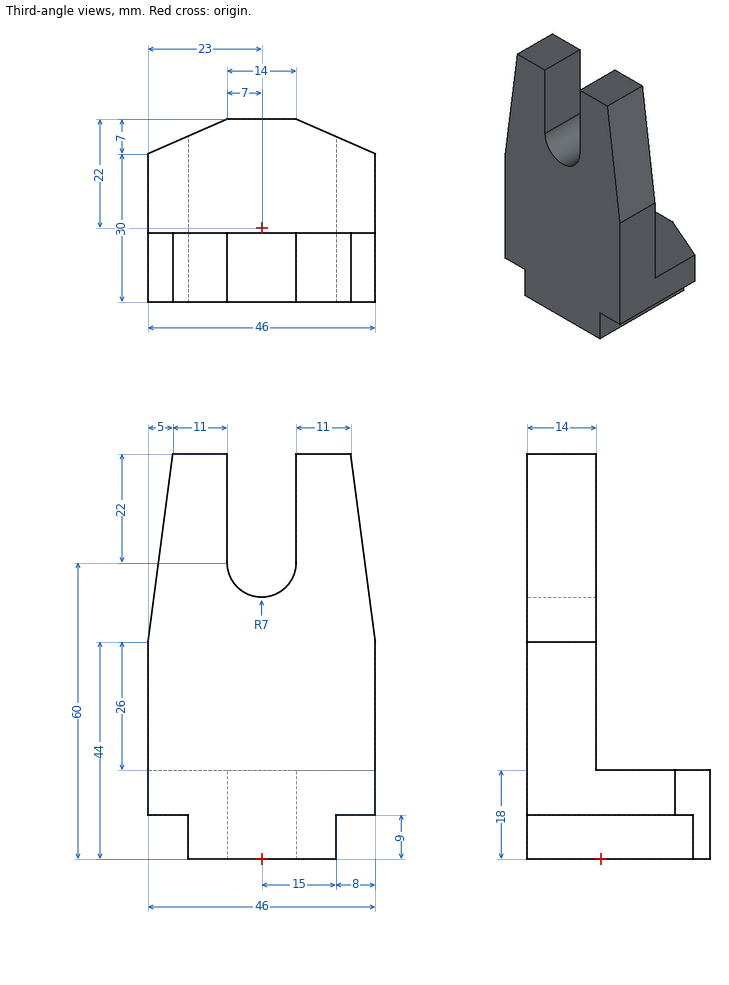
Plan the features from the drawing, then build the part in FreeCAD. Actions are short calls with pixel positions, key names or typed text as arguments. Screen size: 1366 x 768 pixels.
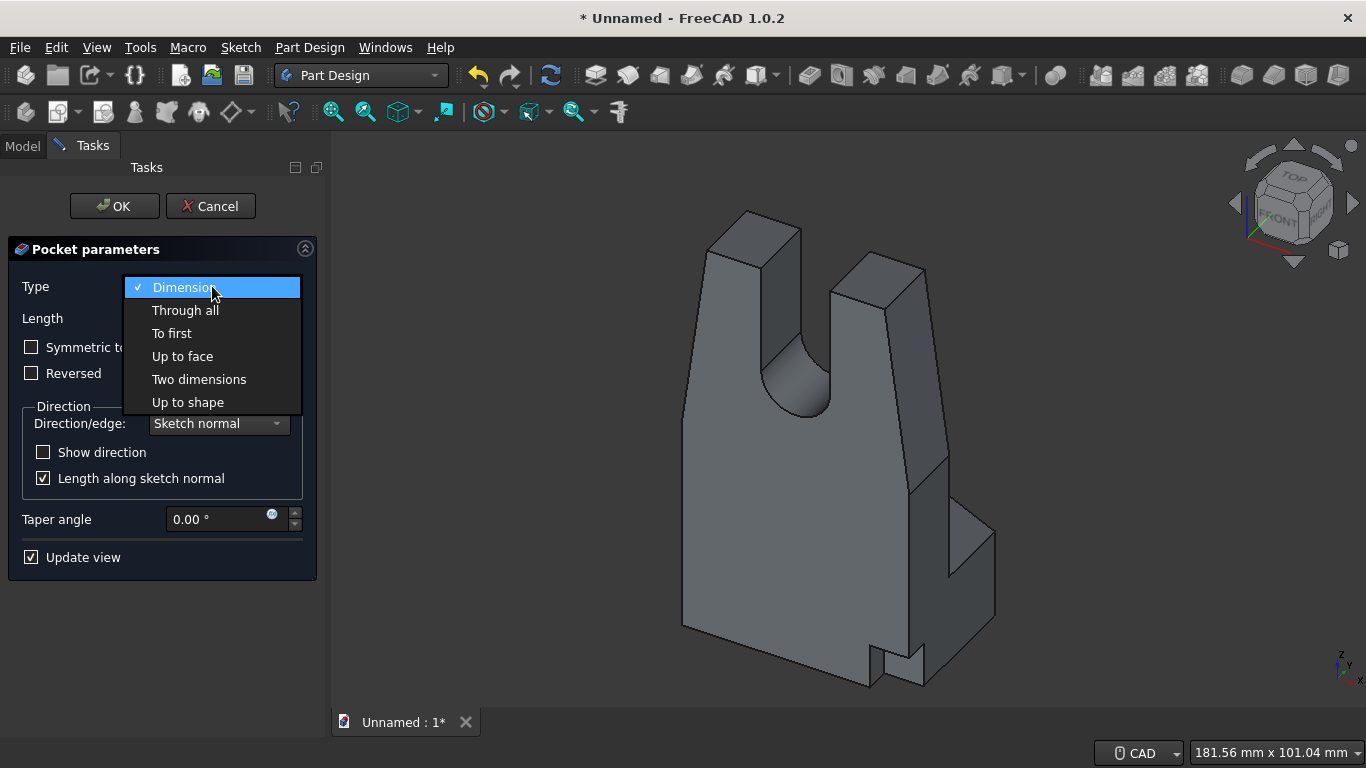
click(212, 310)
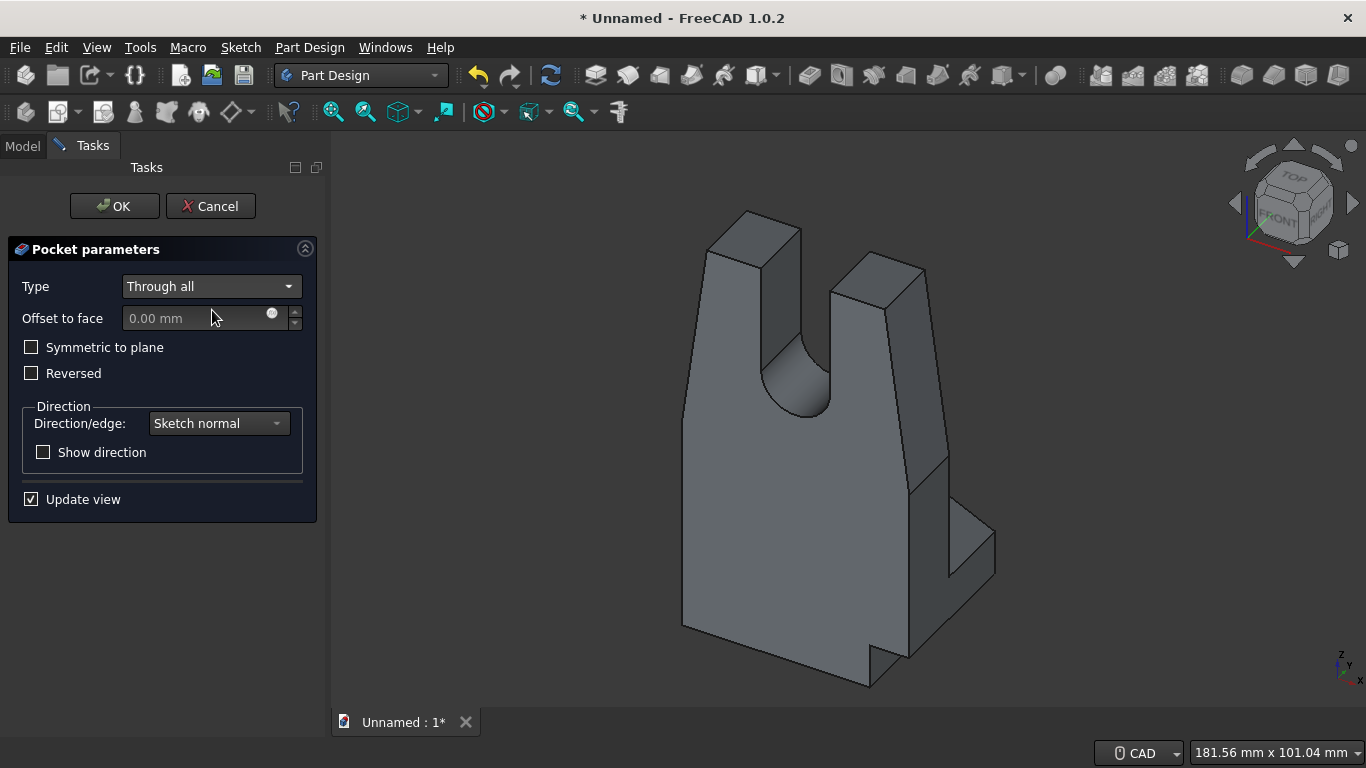
click(115, 206)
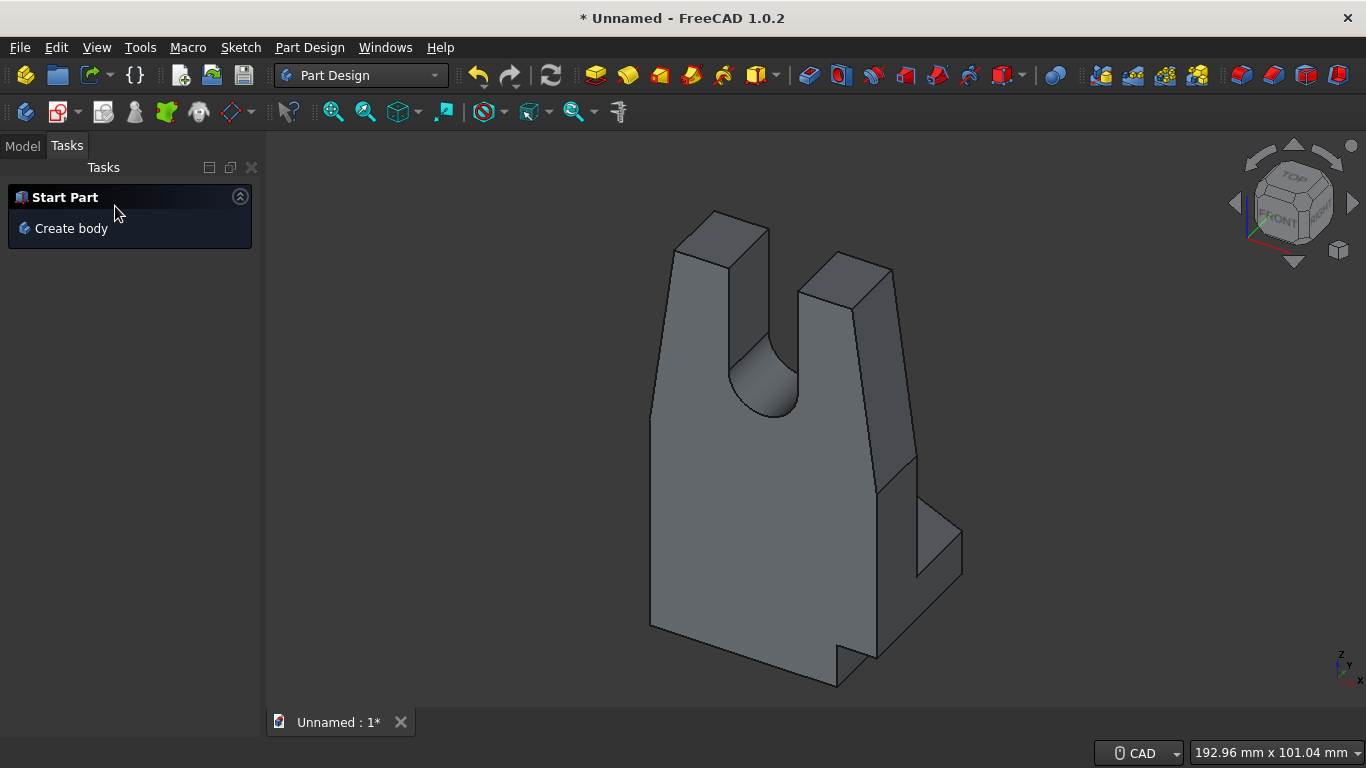
click(23, 145)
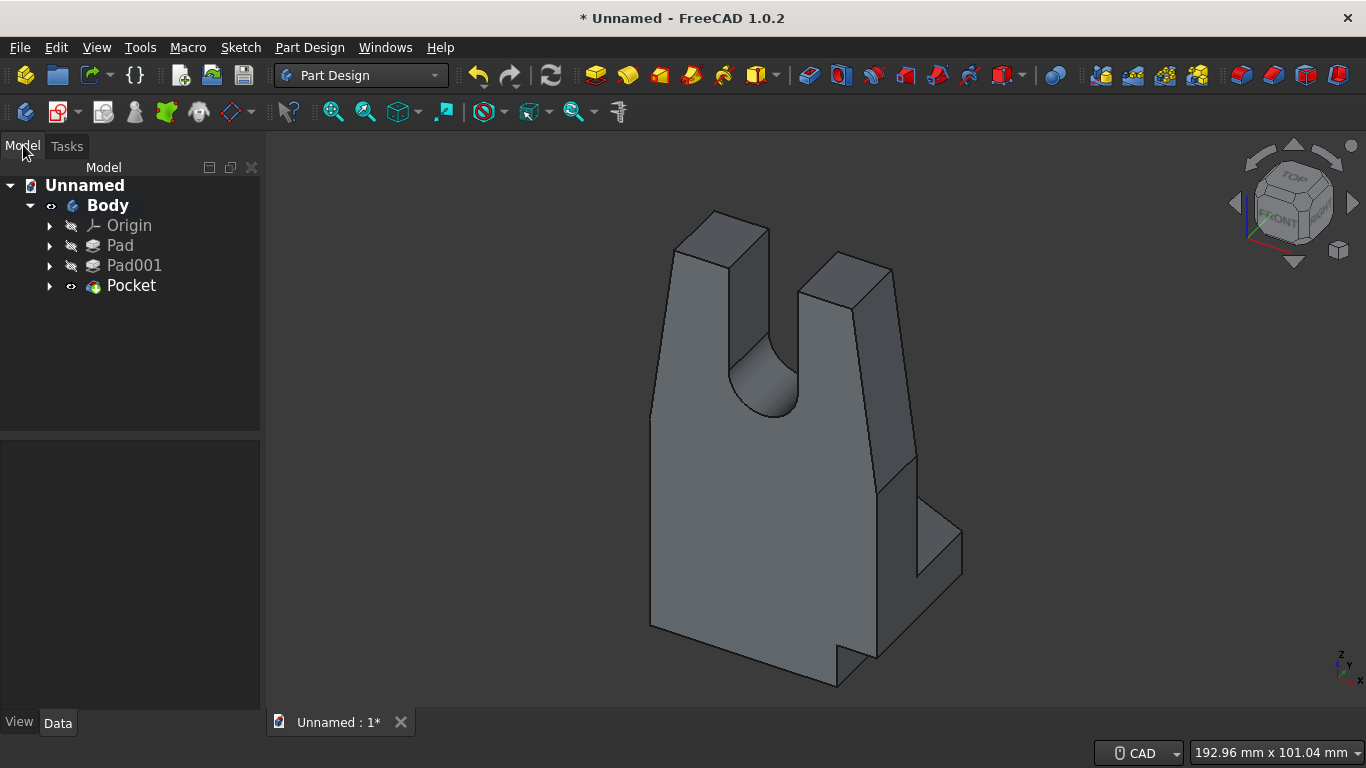
click(116, 286)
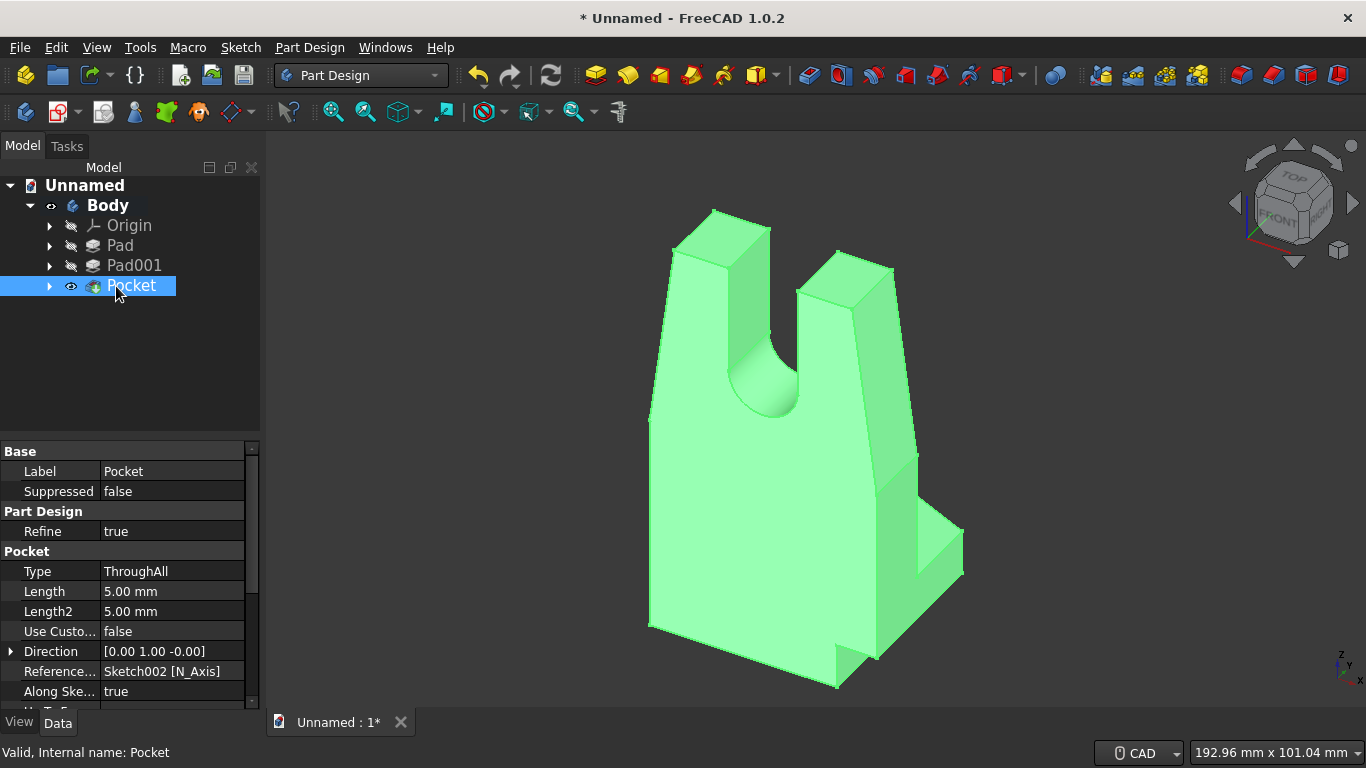
click(1102, 76)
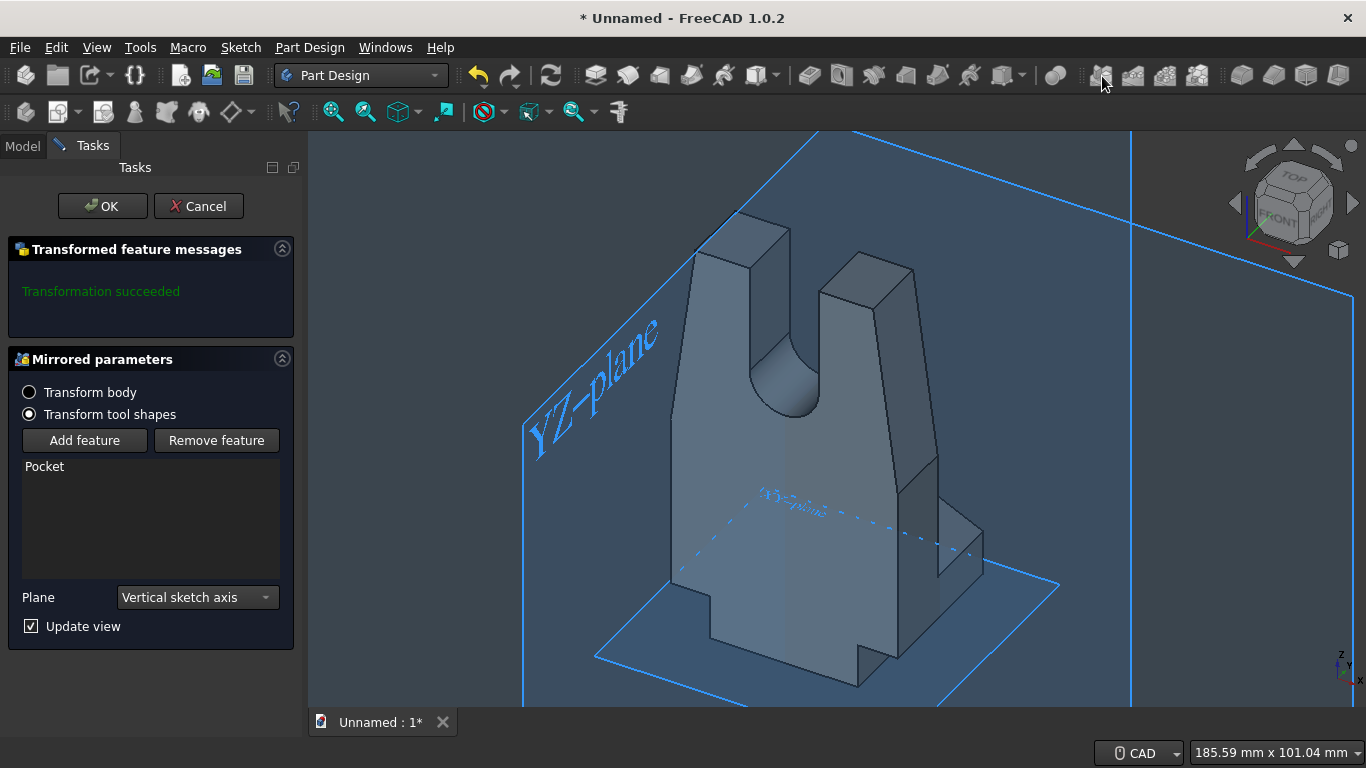
click(198, 598)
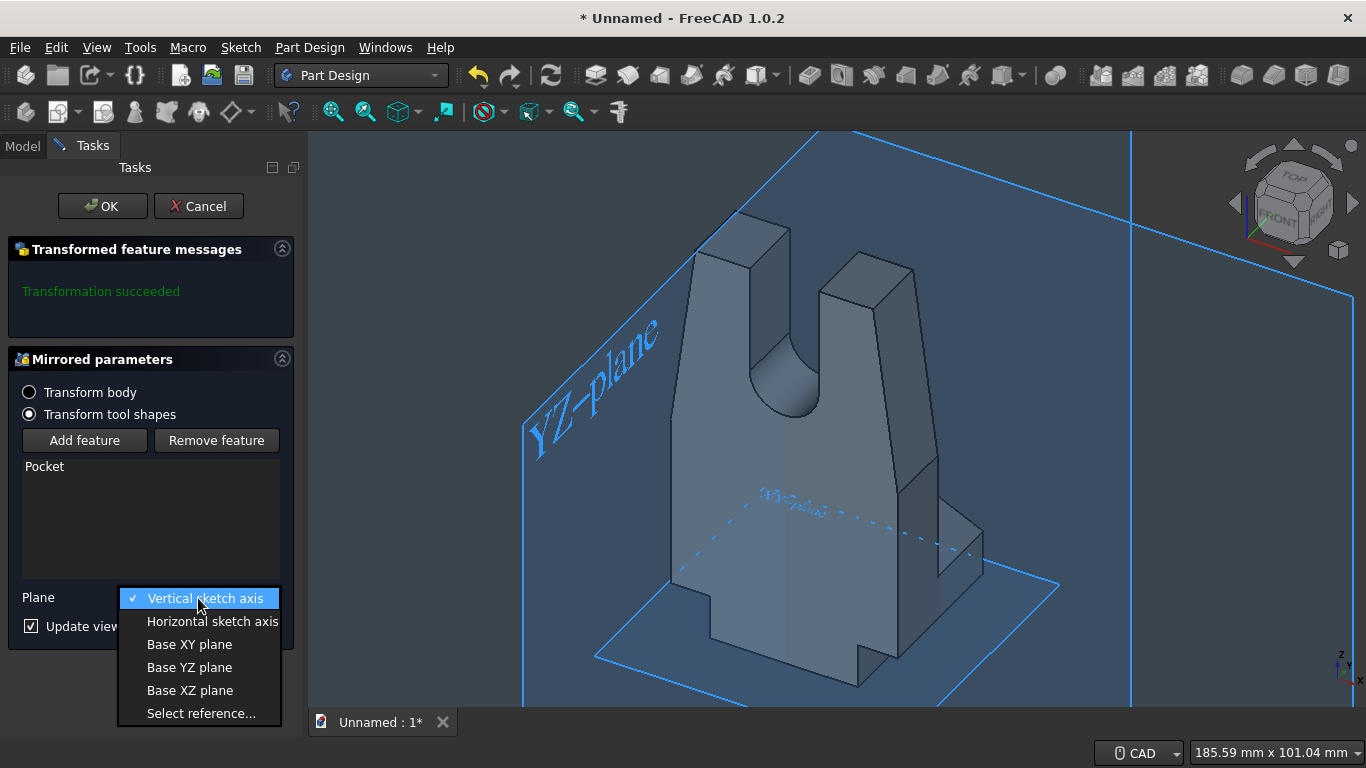
click(198, 668)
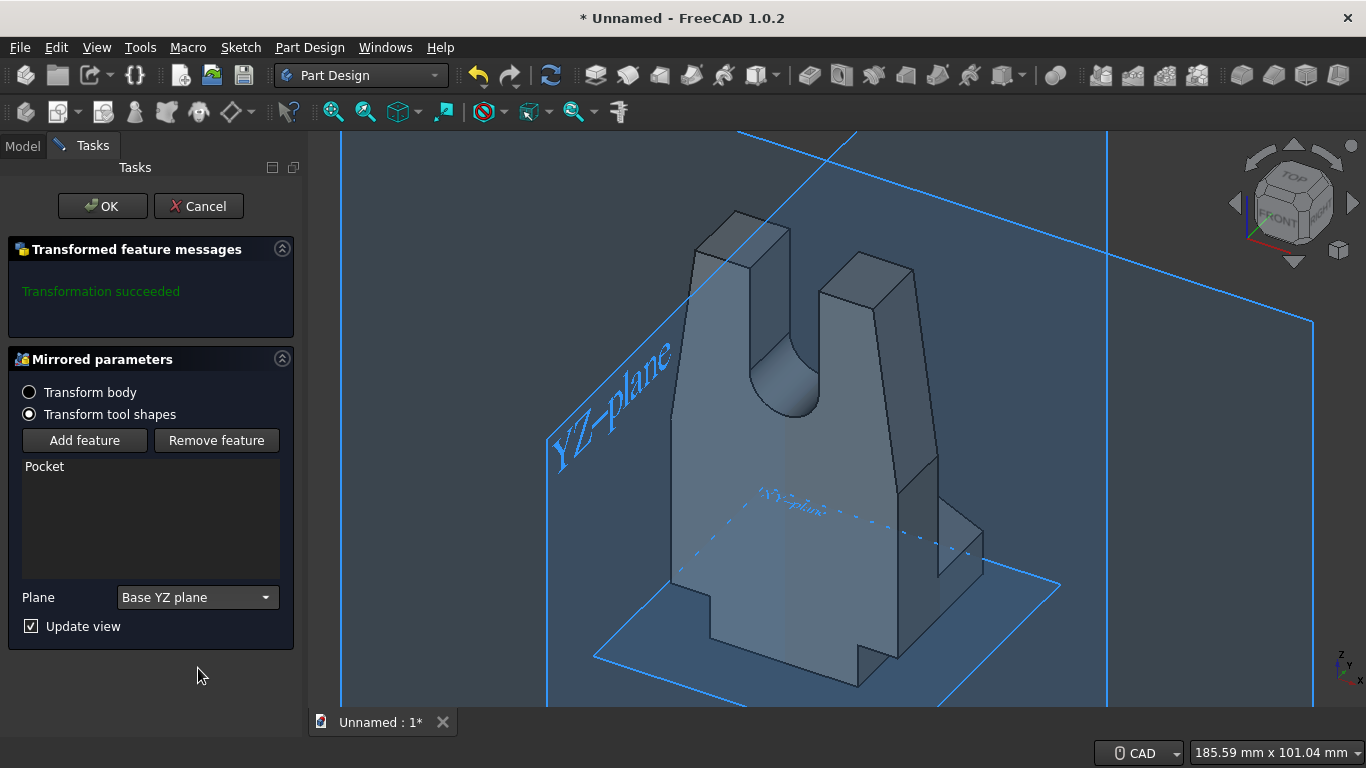
click(103, 206)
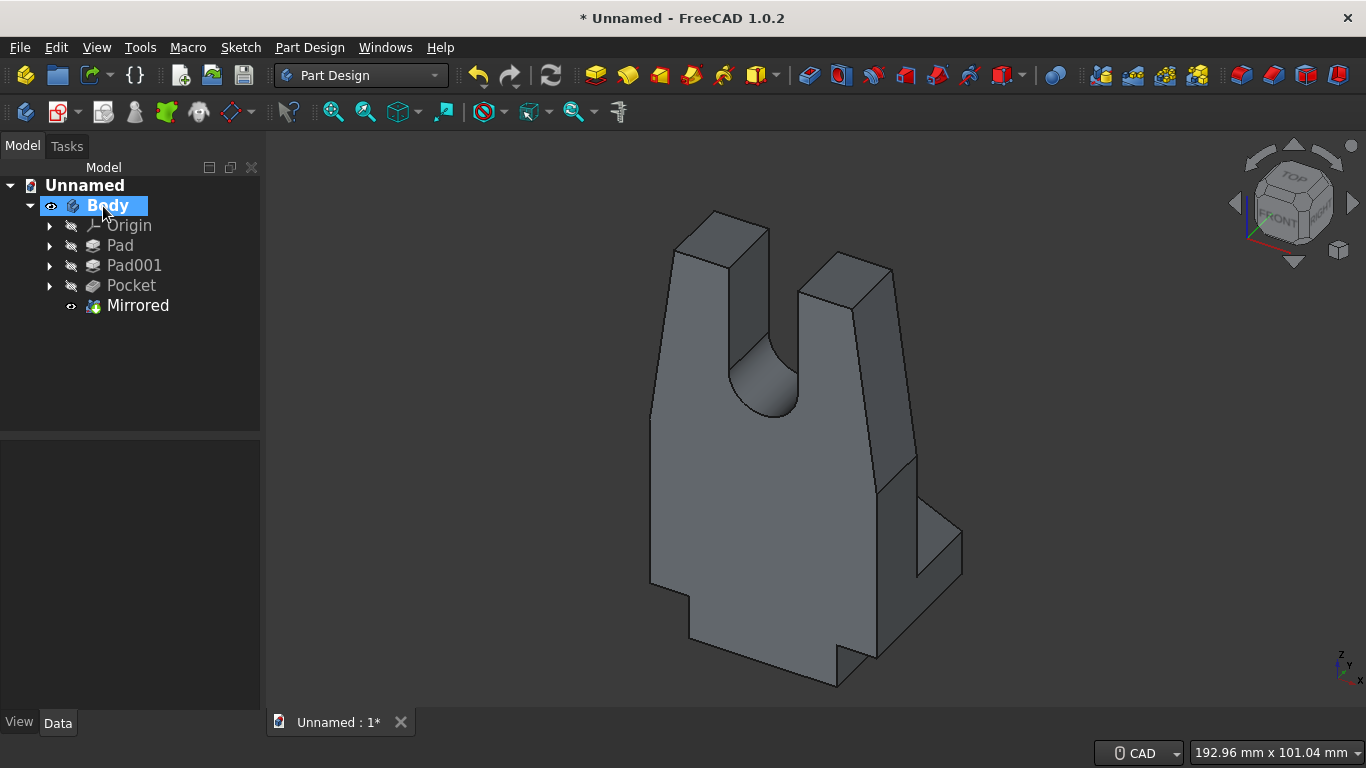
key(0)